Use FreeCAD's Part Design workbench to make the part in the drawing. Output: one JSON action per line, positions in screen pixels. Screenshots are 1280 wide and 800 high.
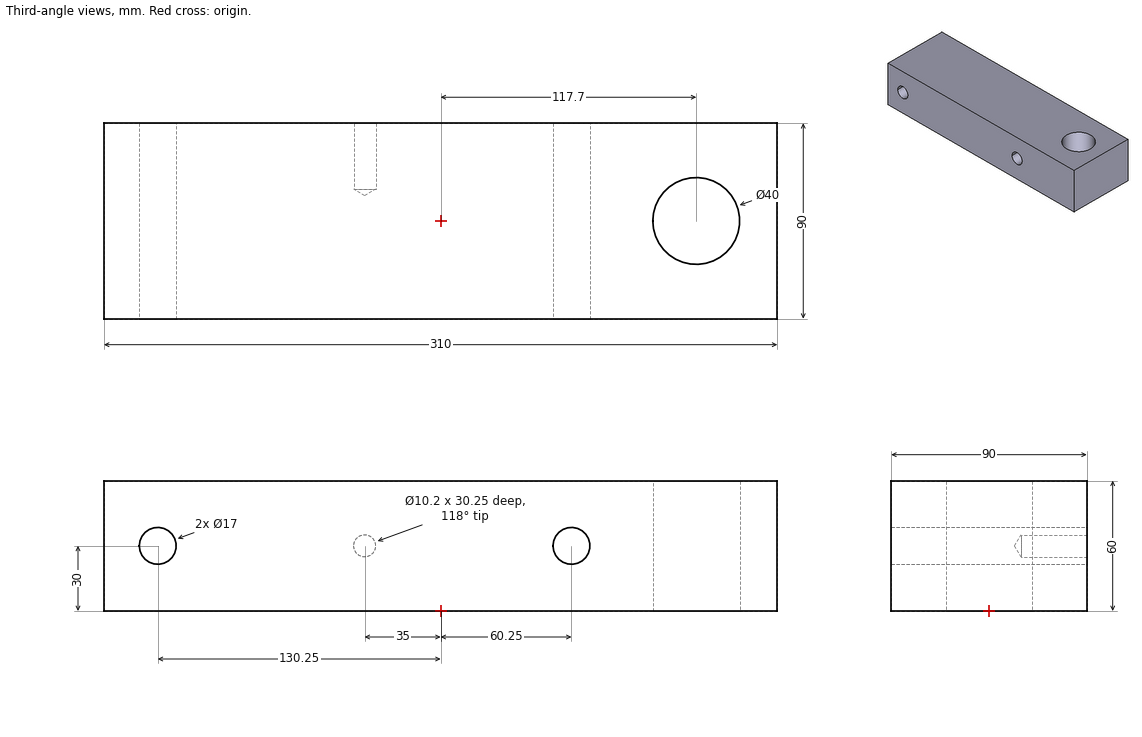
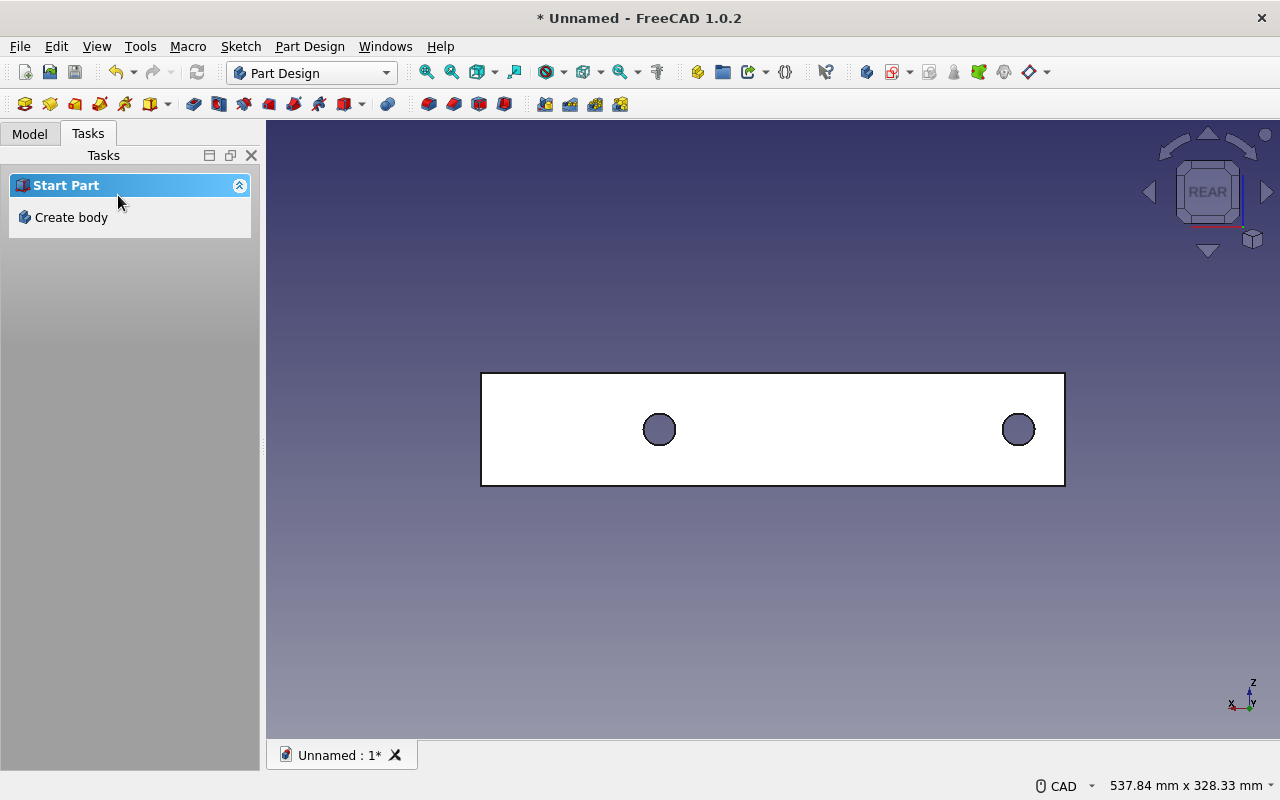
{"action": "left_click", "coordinate": [773, 429]}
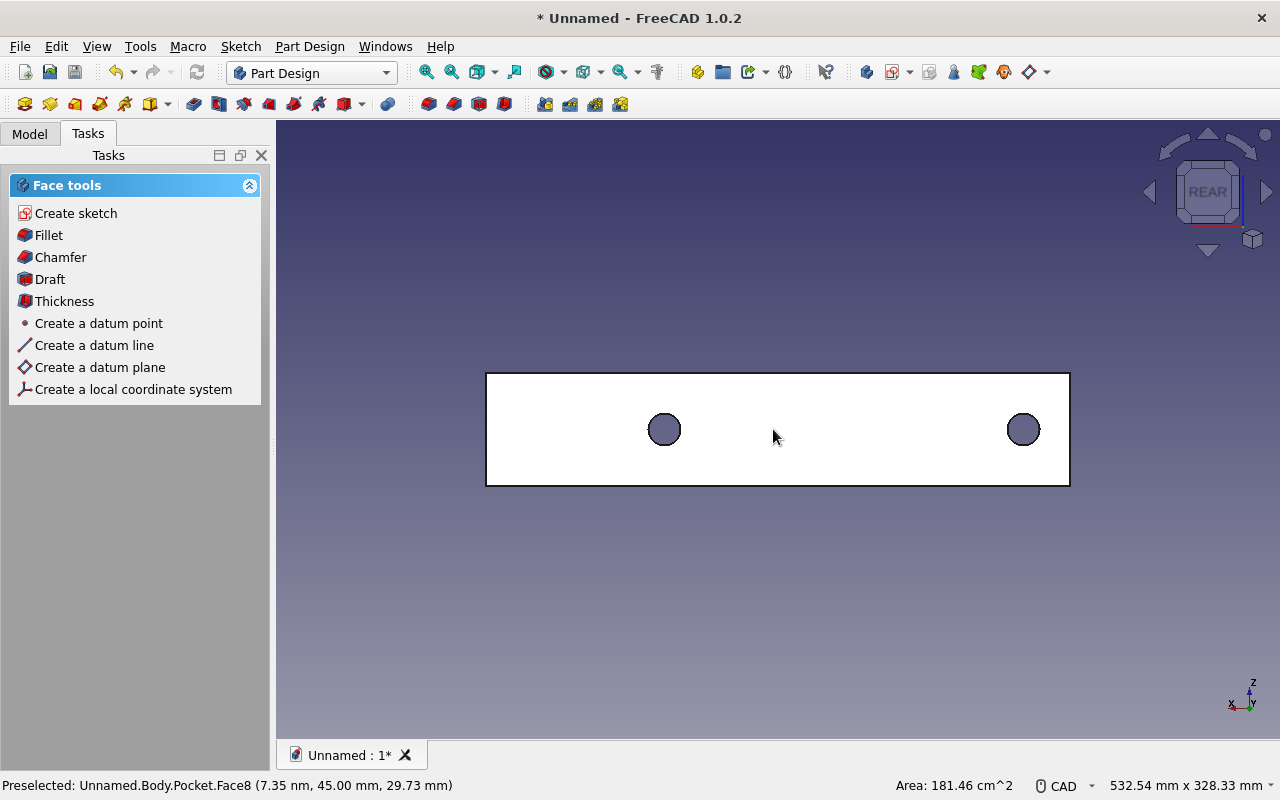
{"action": "left_click", "coordinate": [892, 72]}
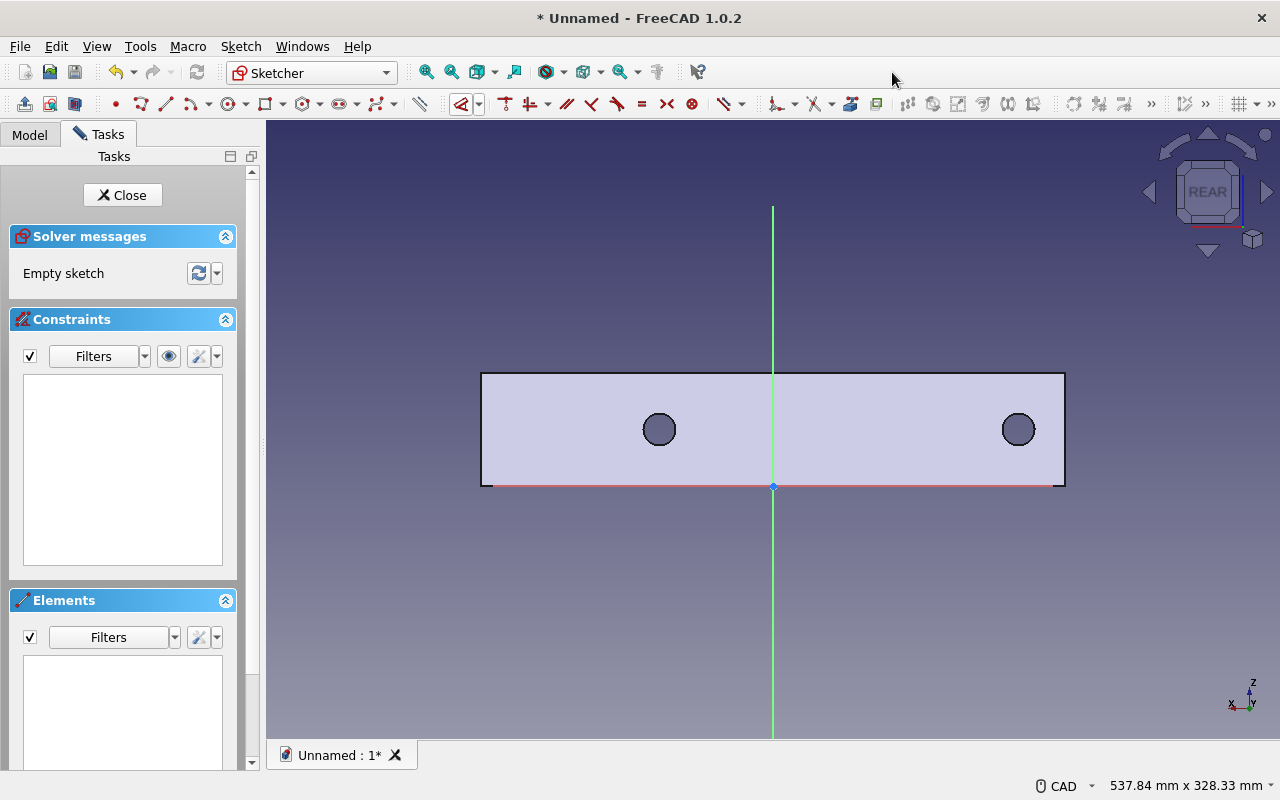
{"action": "scroll", "coordinate": [846, 430], "scroll_direction": "up", "scroll_amount": 15}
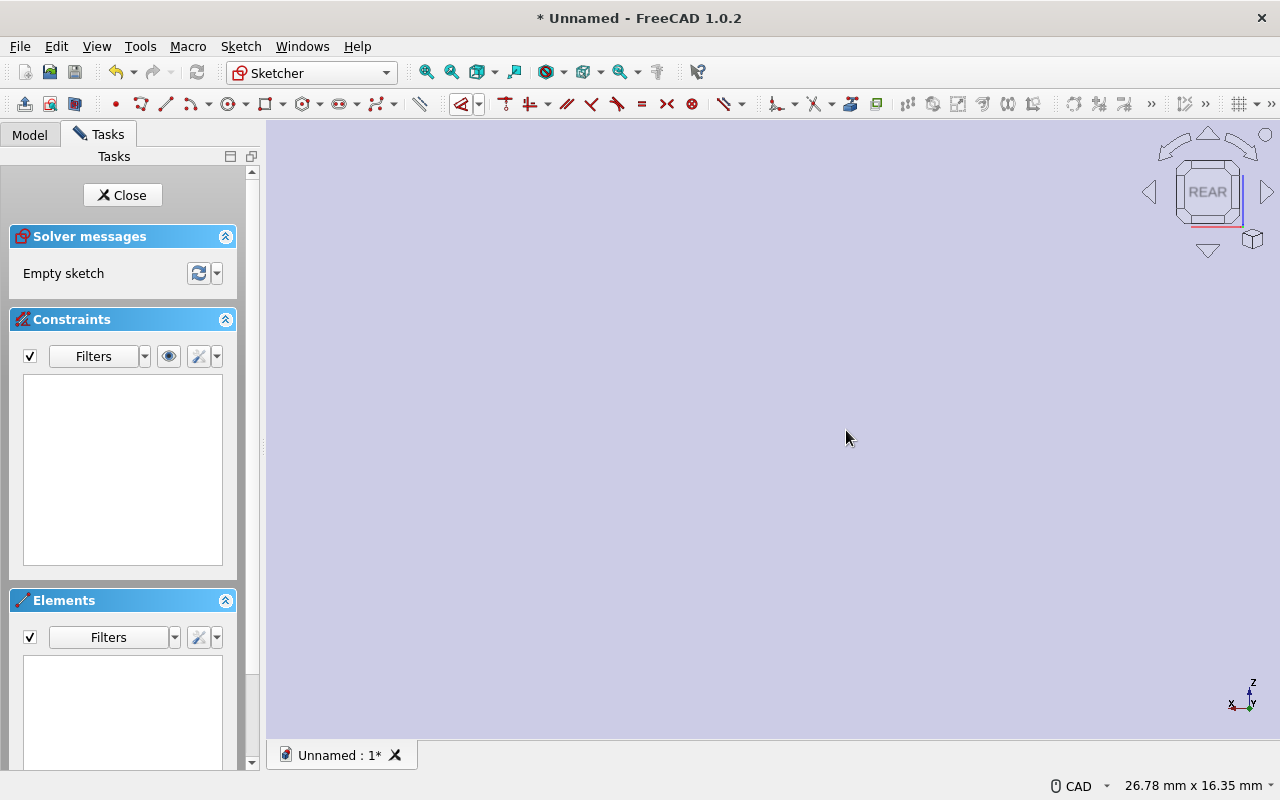
{"action": "left_click", "coordinate": [228, 104]}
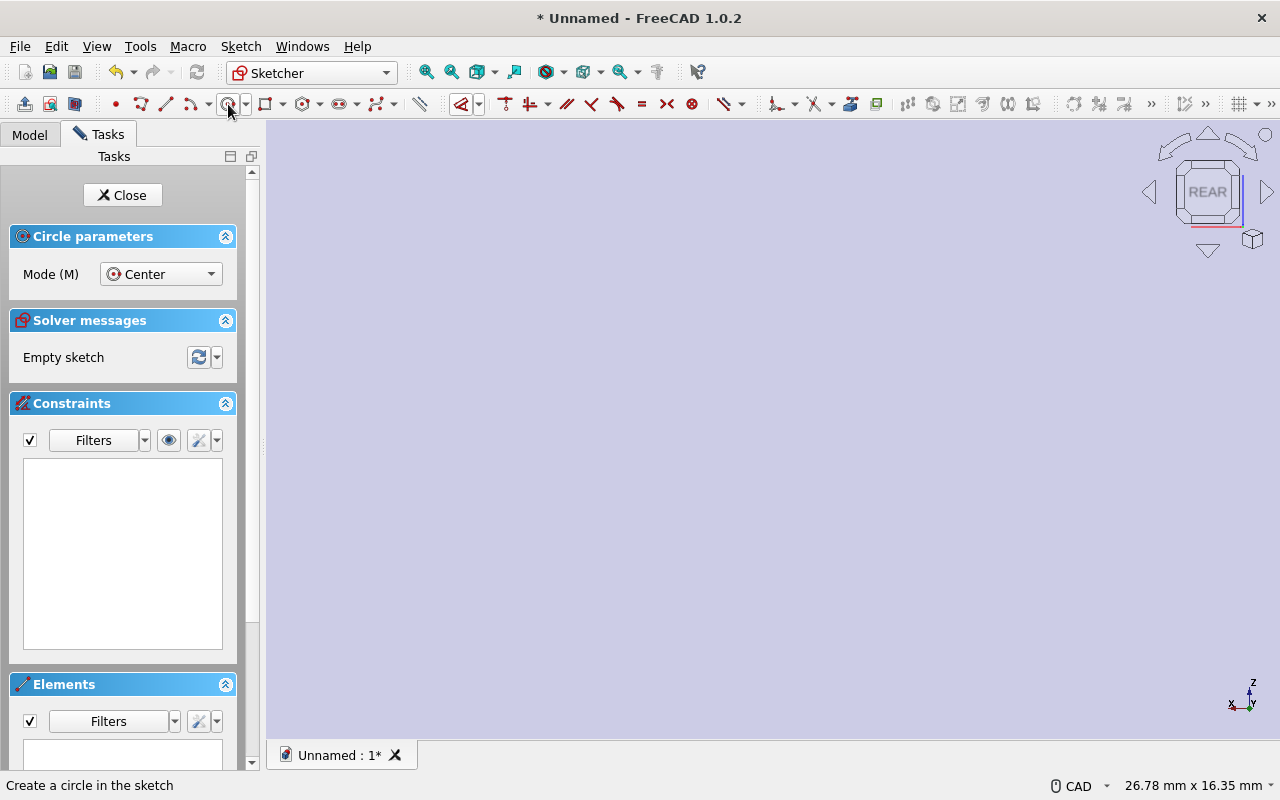
{"action": "left_click", "coordinate": [694, 410]}
{"action": "left_click", "coordinate": [831, 274]}
{"action": "key", "text": "Escape"}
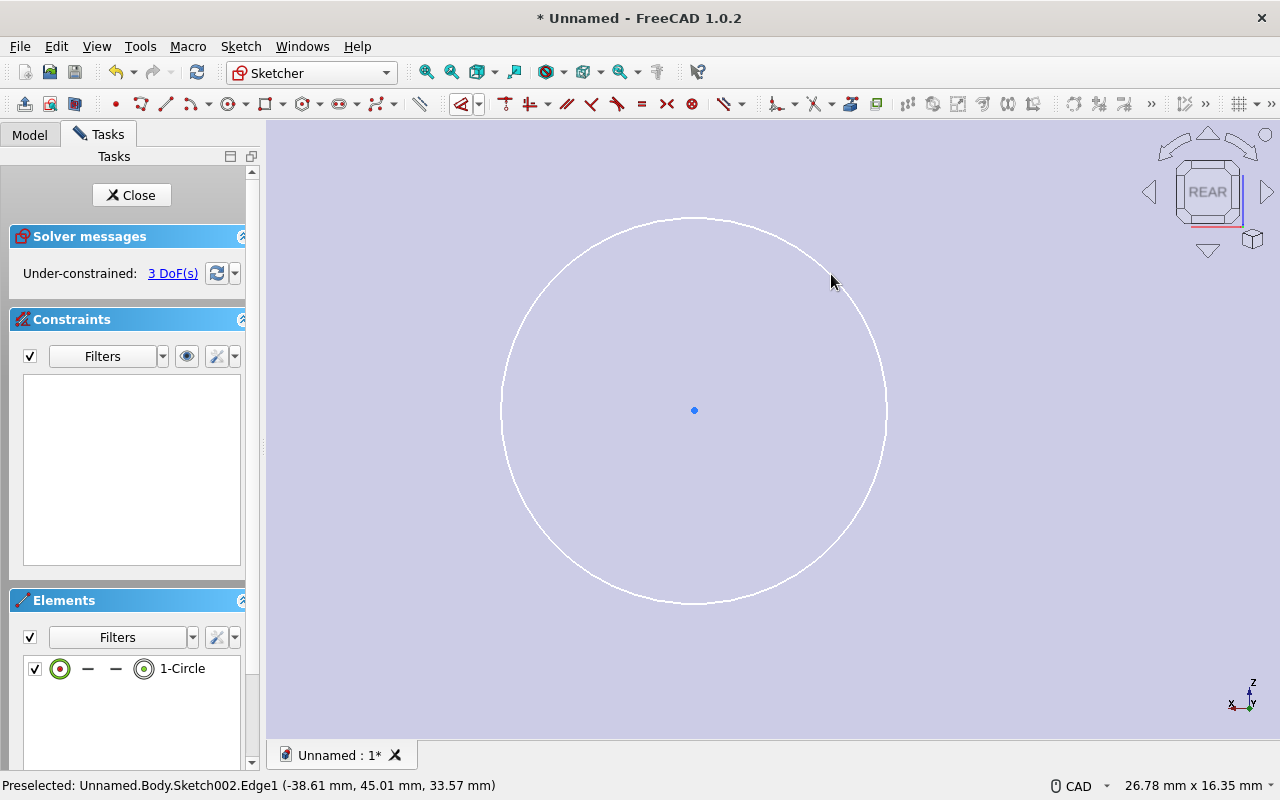
{"action": "left_click", "coordinate": [830, 274]}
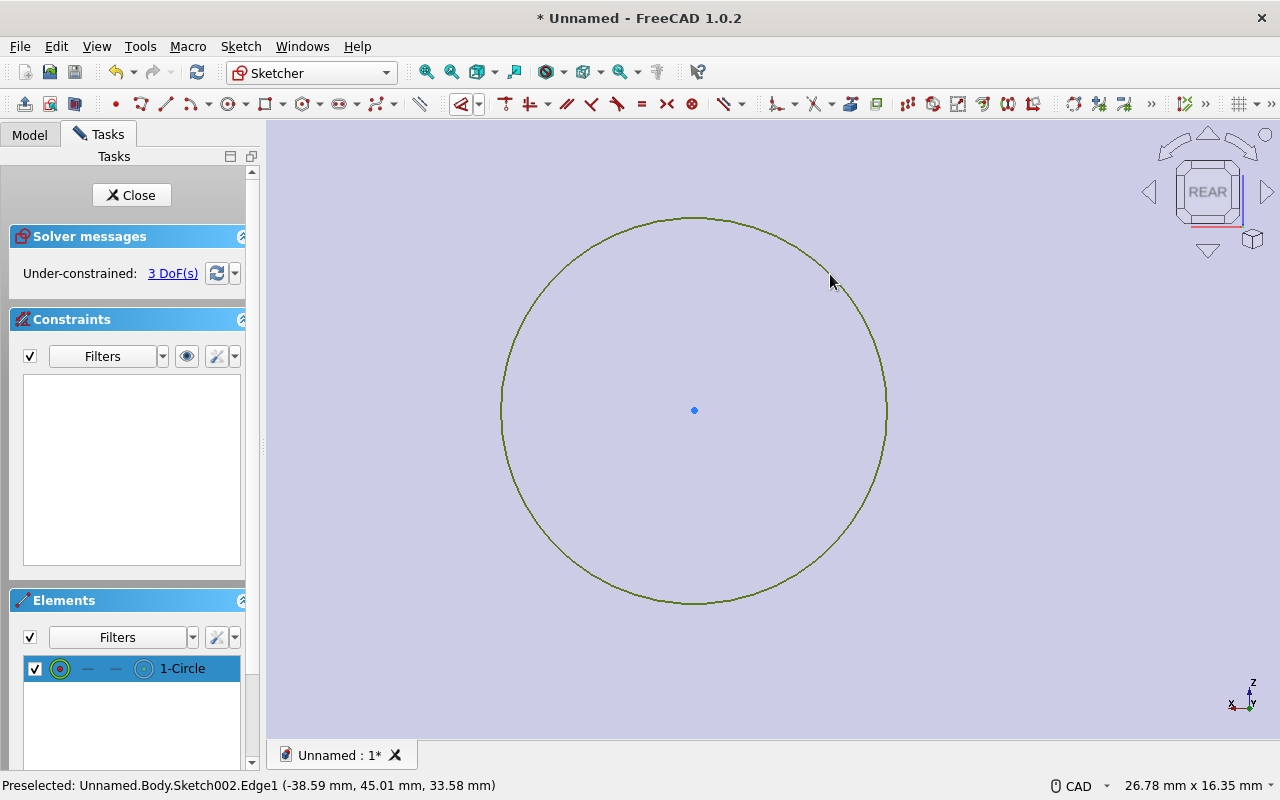
{"action": "left_click", "coordinate": [478, 104]}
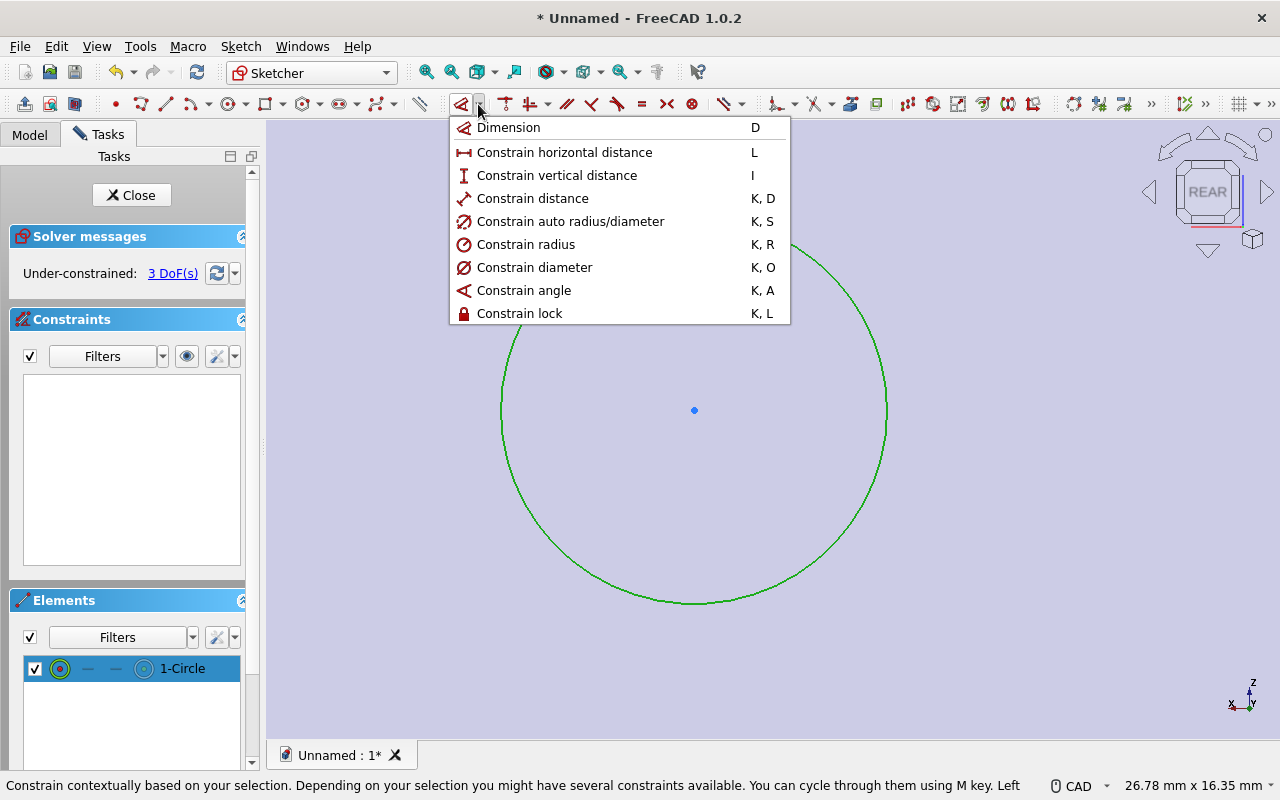
{"action": "left_click", "coordinate": [620, 268]}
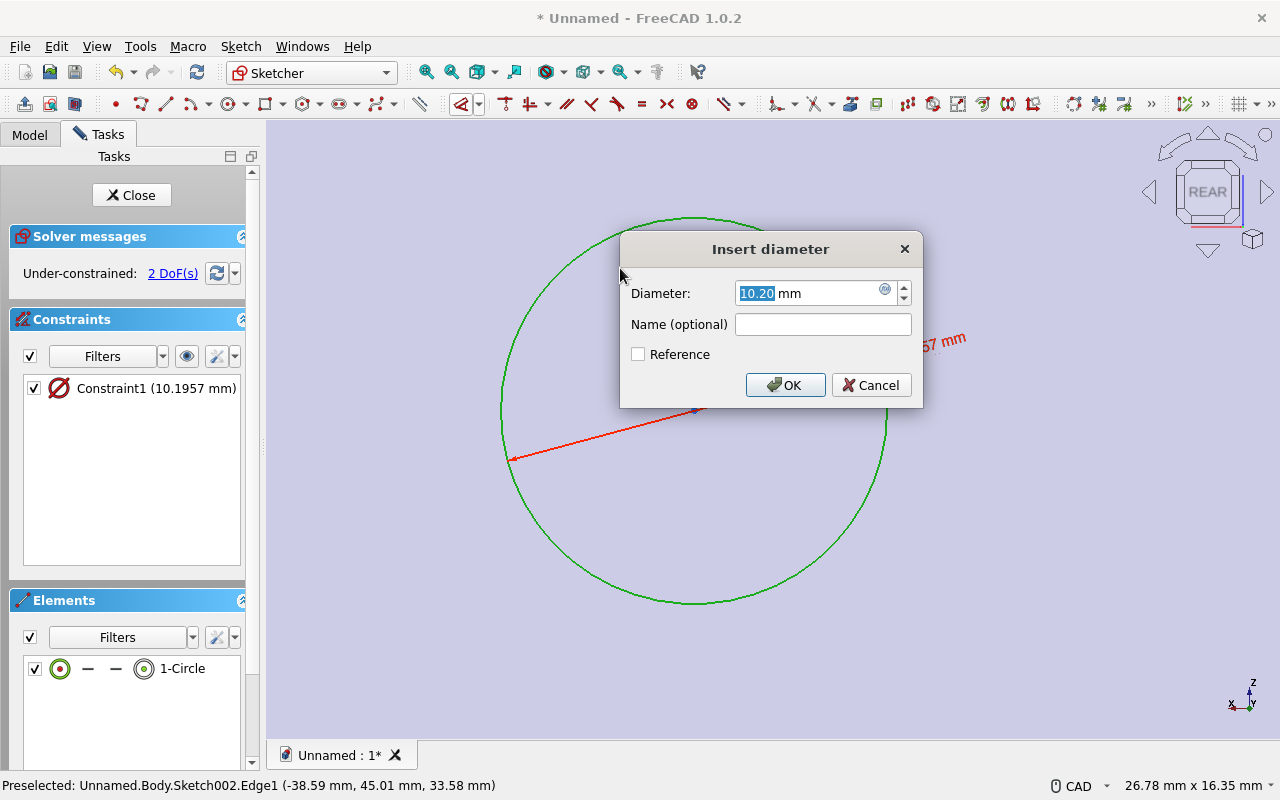
{"action": "type", "text": "10.2"}
{"action": "key", "text": "Return"}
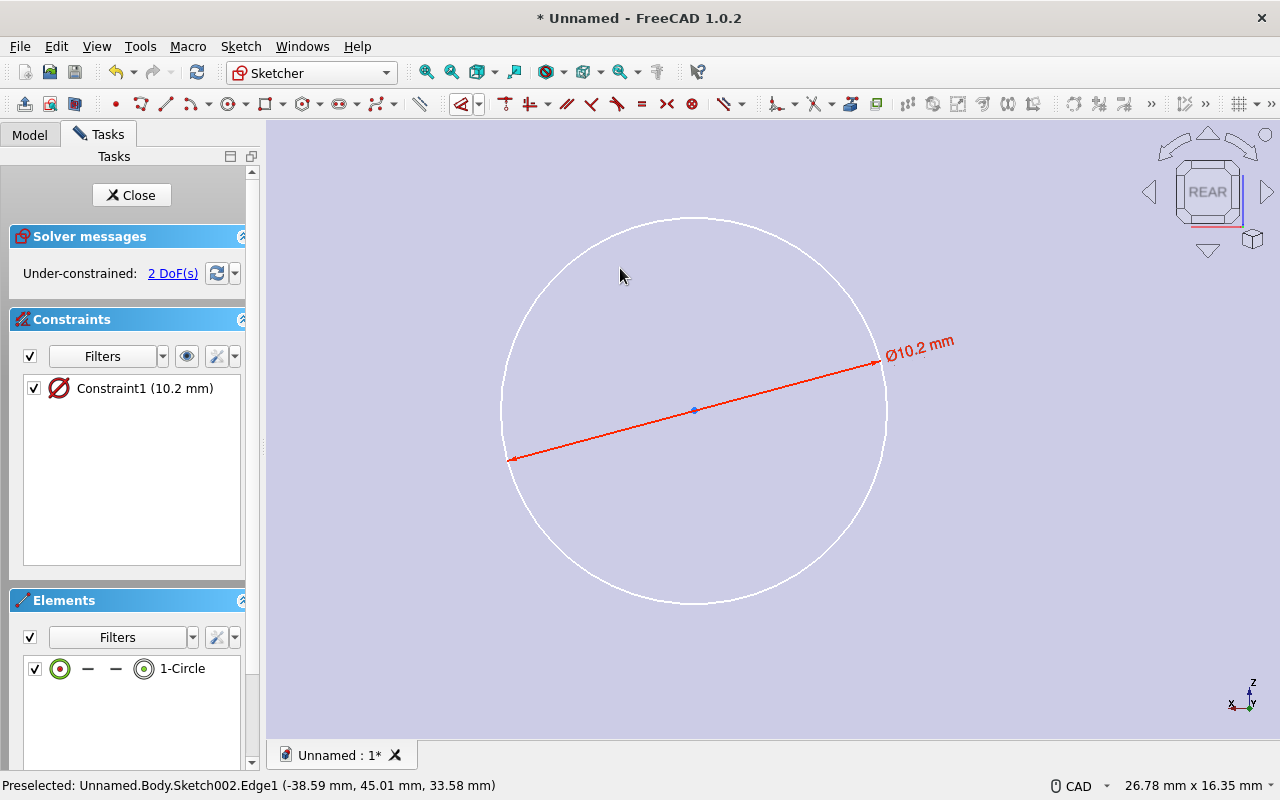
{"action": "left_click", "coordinate": [694, 411]}